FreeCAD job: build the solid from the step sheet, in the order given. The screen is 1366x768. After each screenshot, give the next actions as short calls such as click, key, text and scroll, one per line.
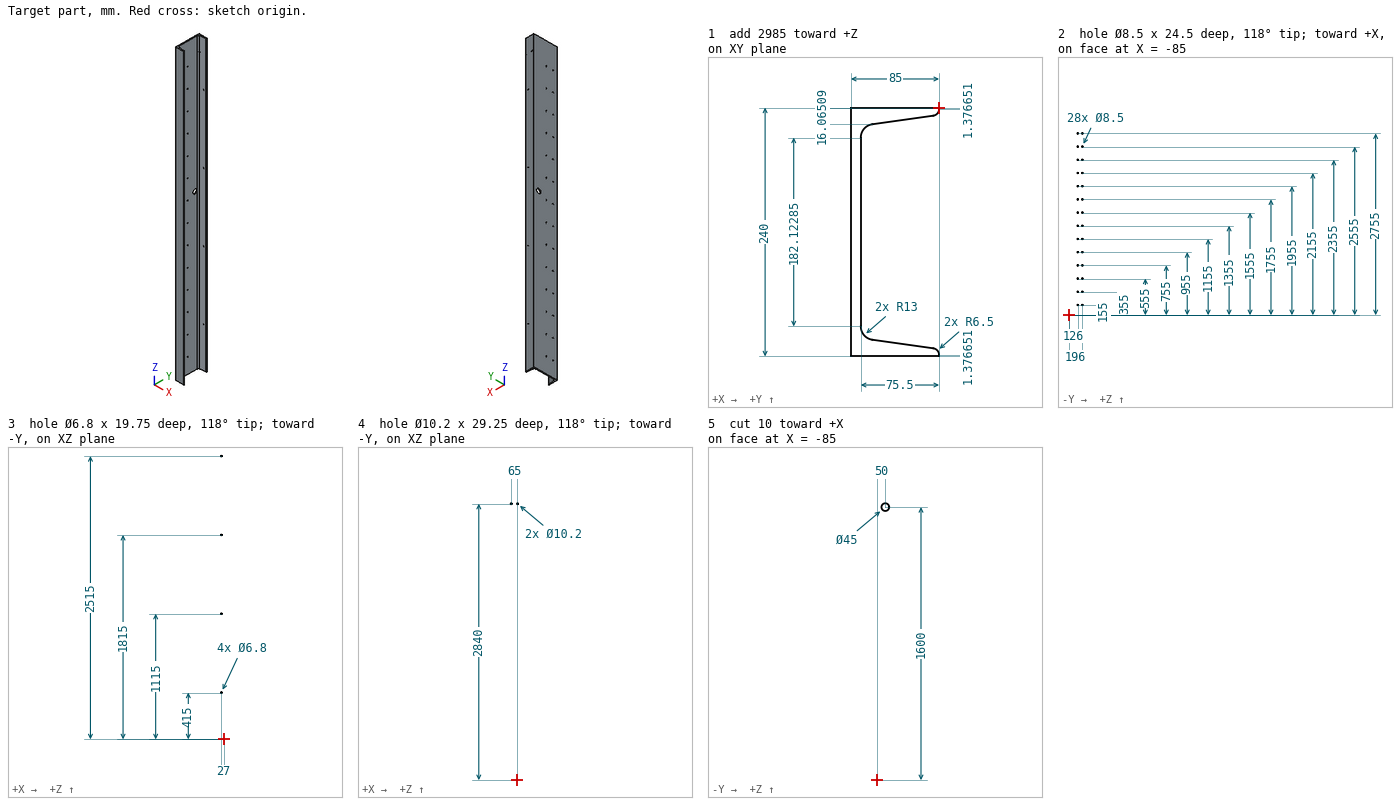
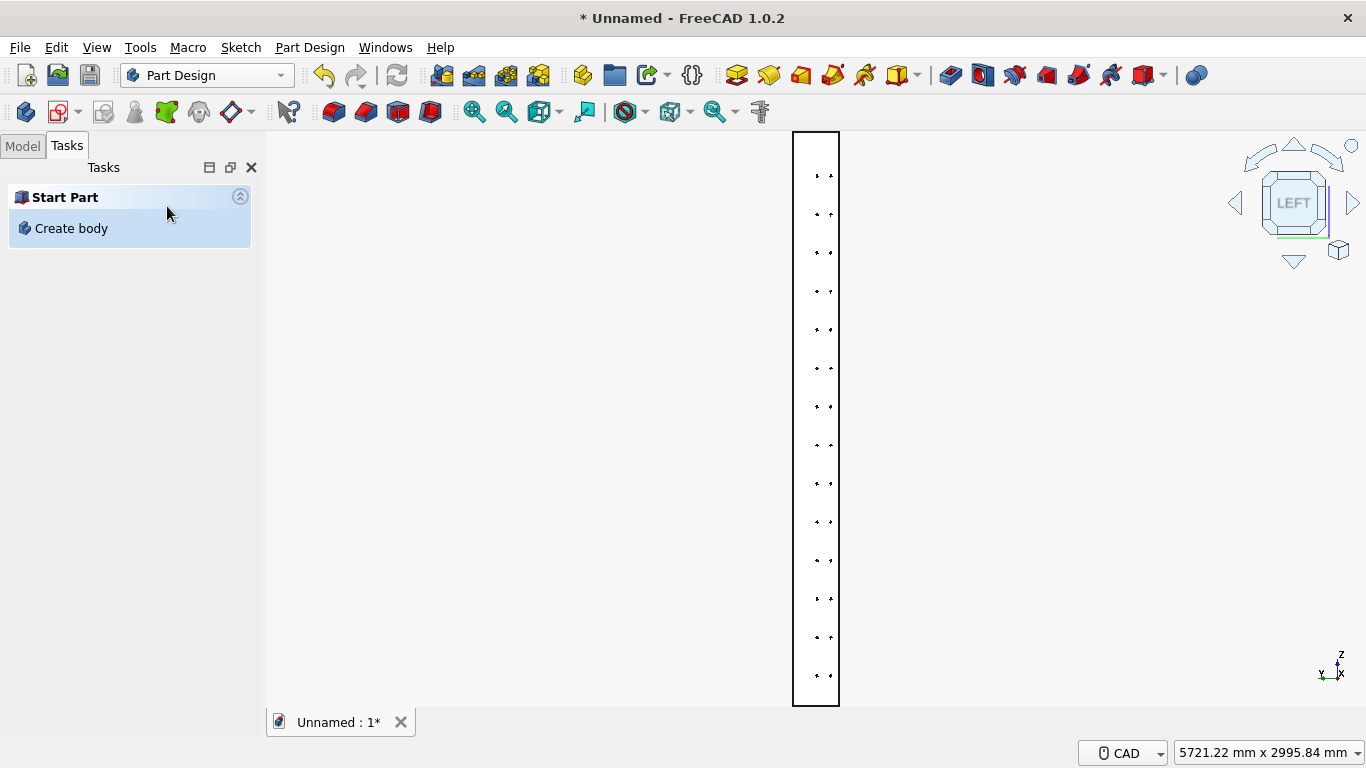
click(58, 112)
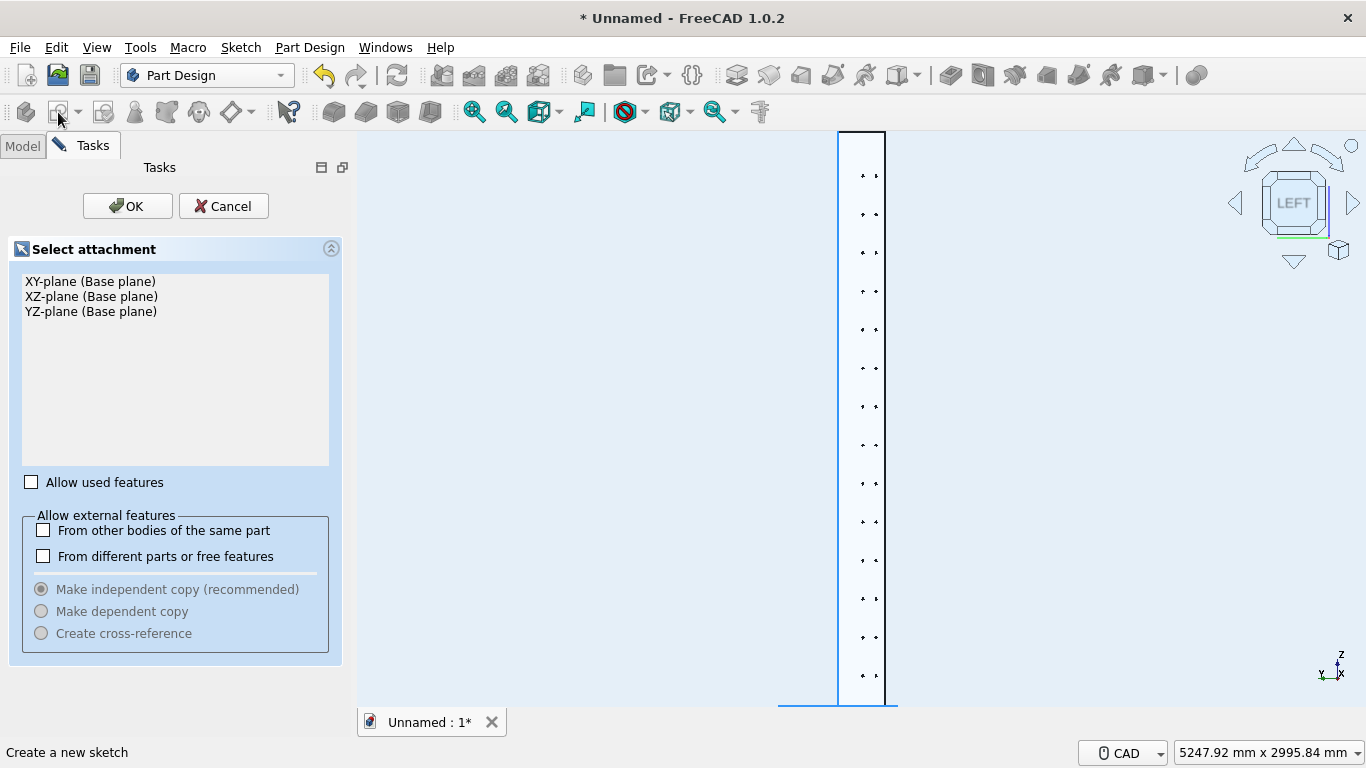
click(82, 296)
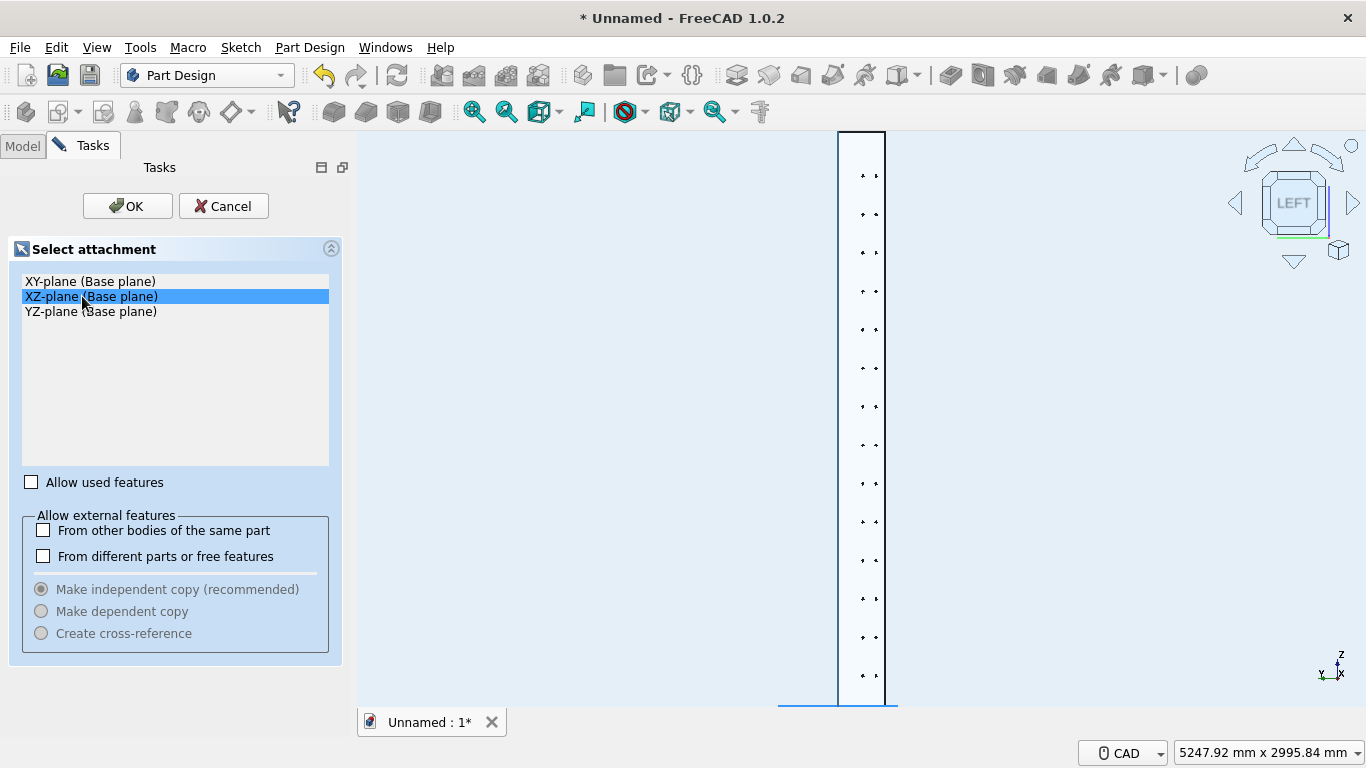
click(128, 206)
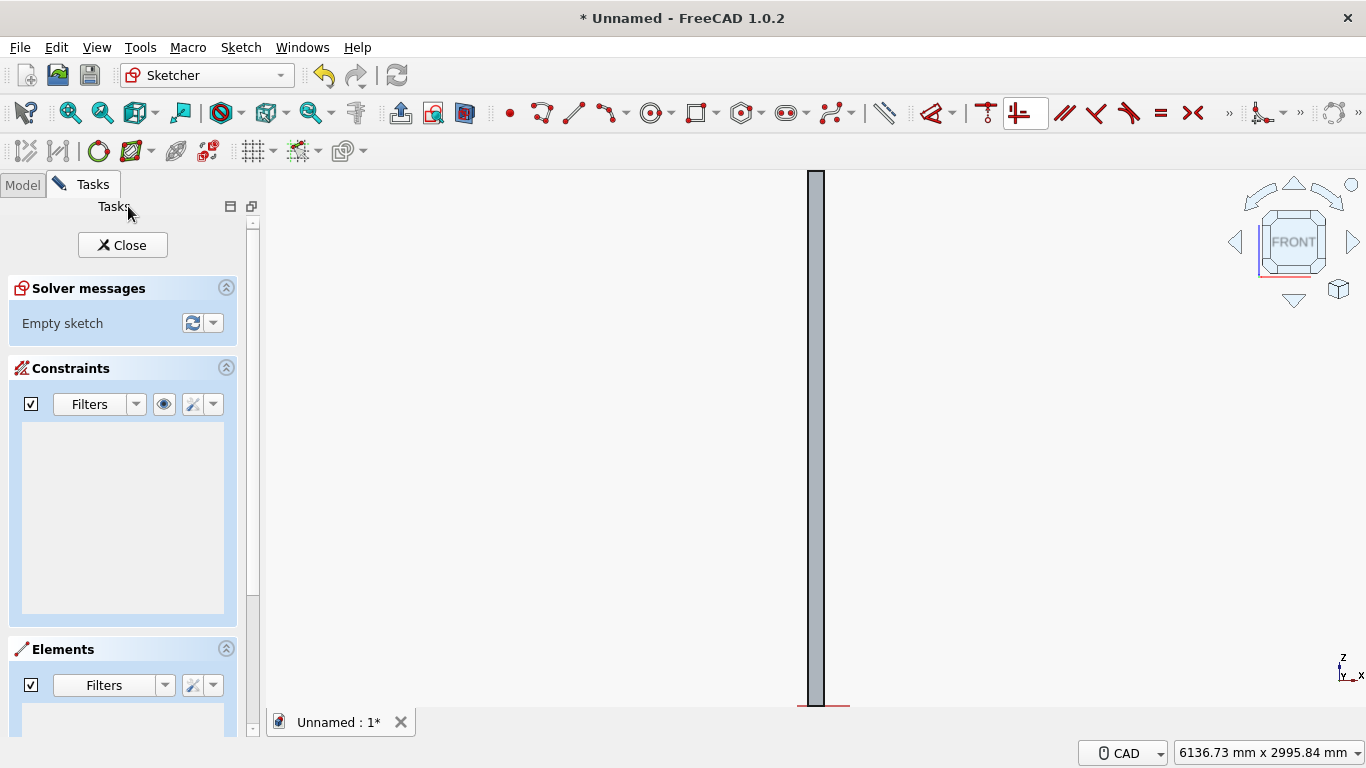
click(466, 114)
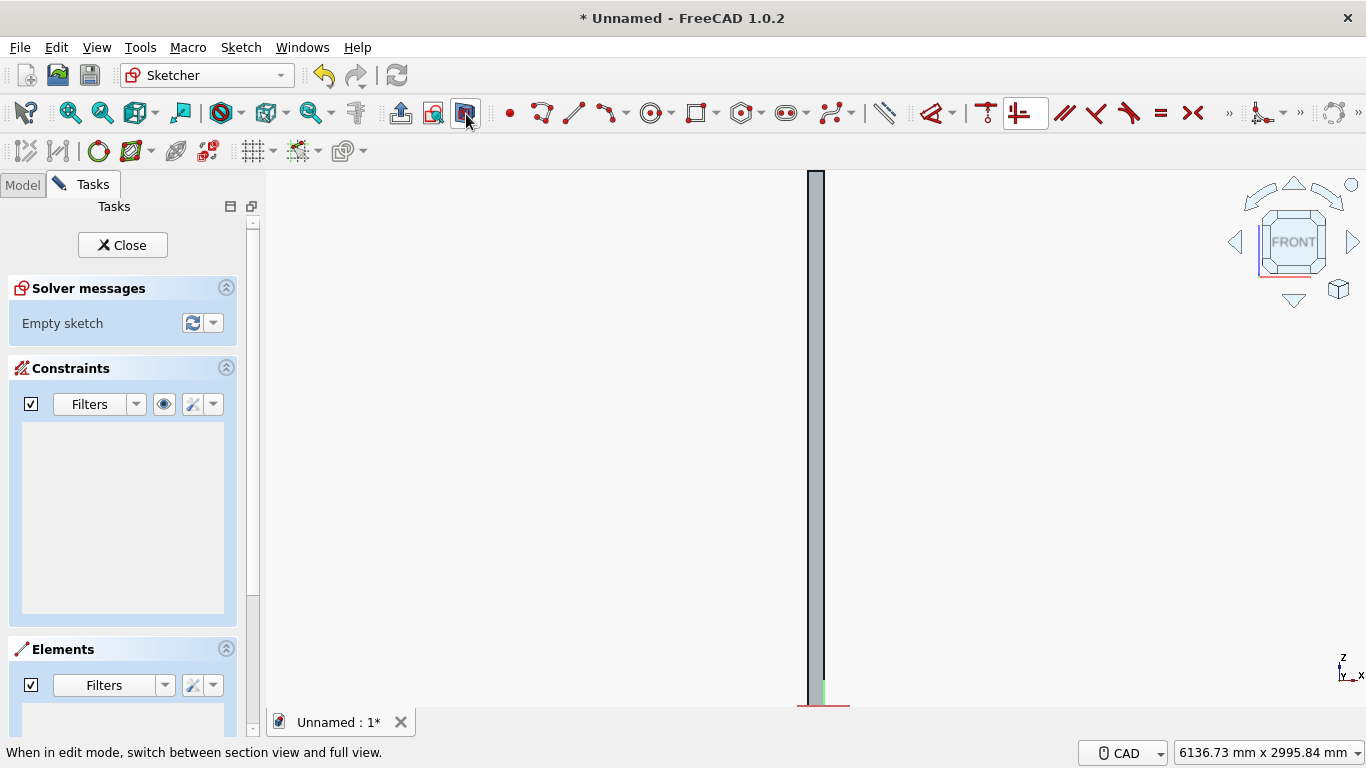
scroll(416, 250, down, 1)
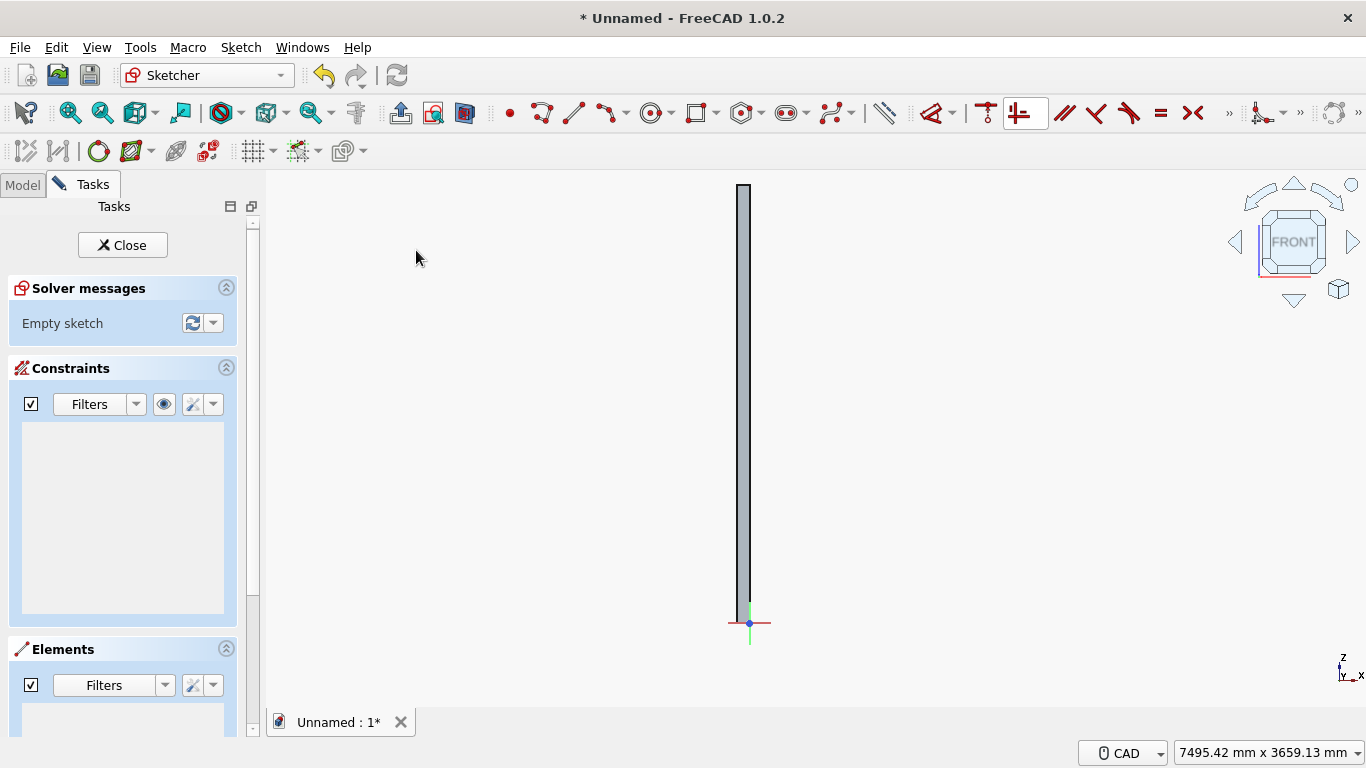
click(652, 114)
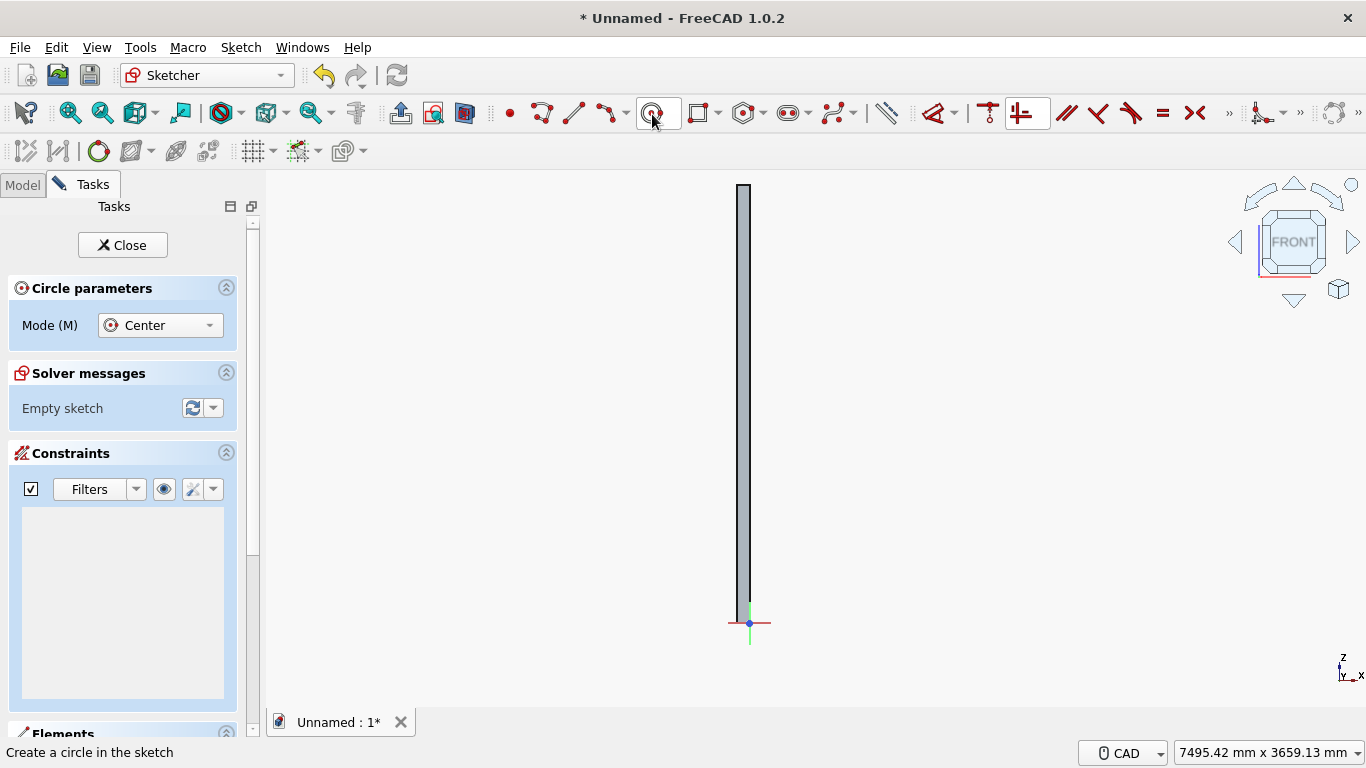
scroll(746, 562, up, 20)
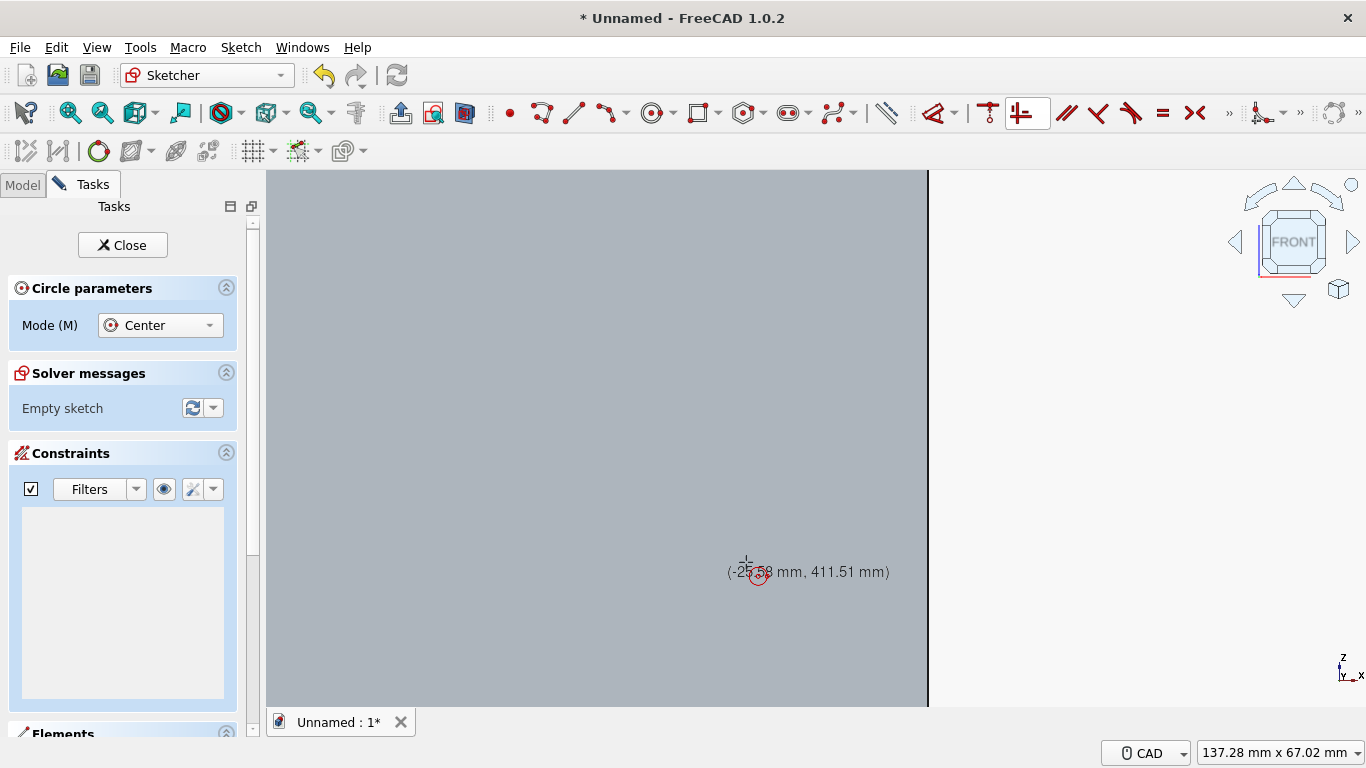
scroll(748, 438, down, 15)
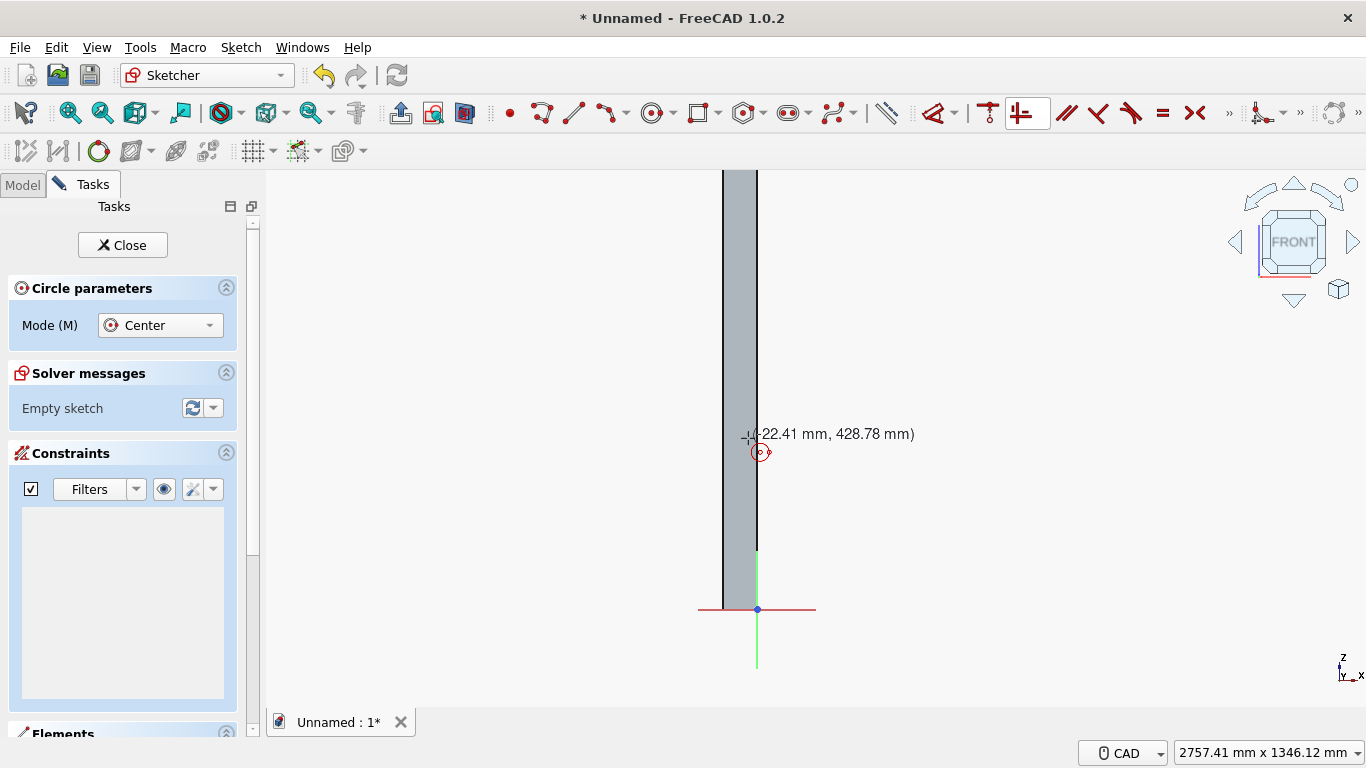
scroll(745, 631, down, 5)